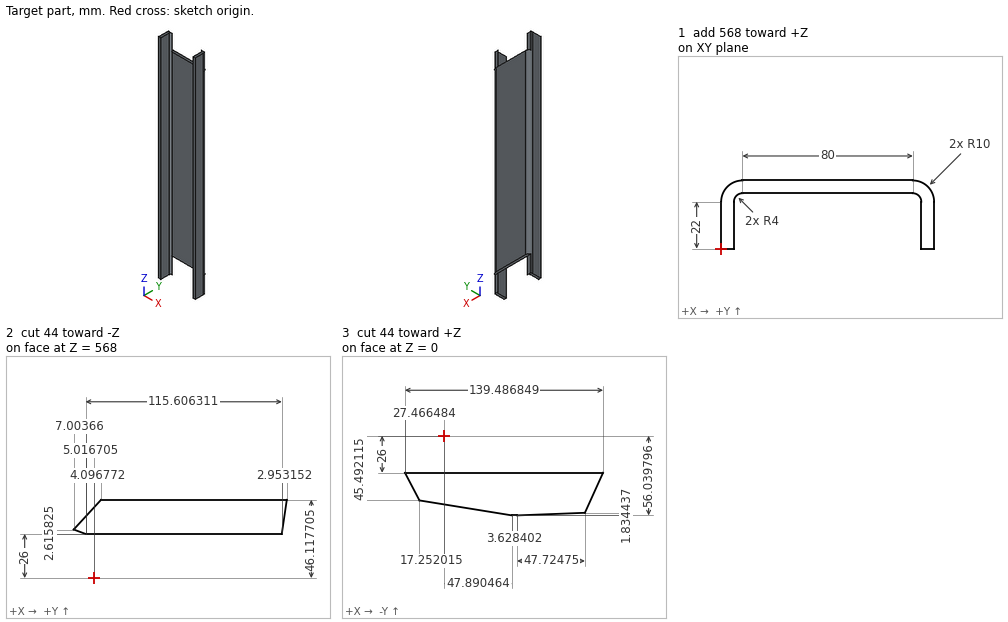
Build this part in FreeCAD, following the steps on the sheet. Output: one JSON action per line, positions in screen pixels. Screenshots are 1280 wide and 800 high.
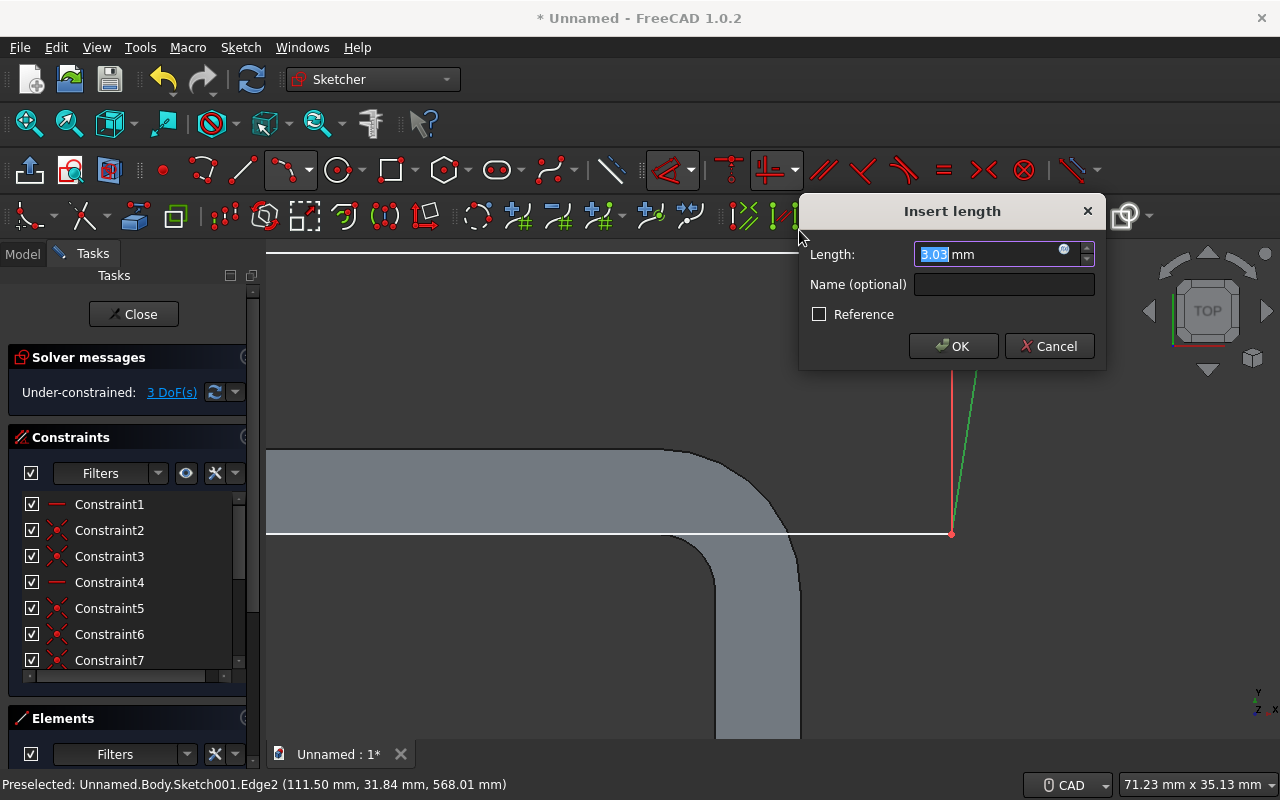
{"action": "type", "text": "2.953152"}
{"action": "key", "text": "Return"}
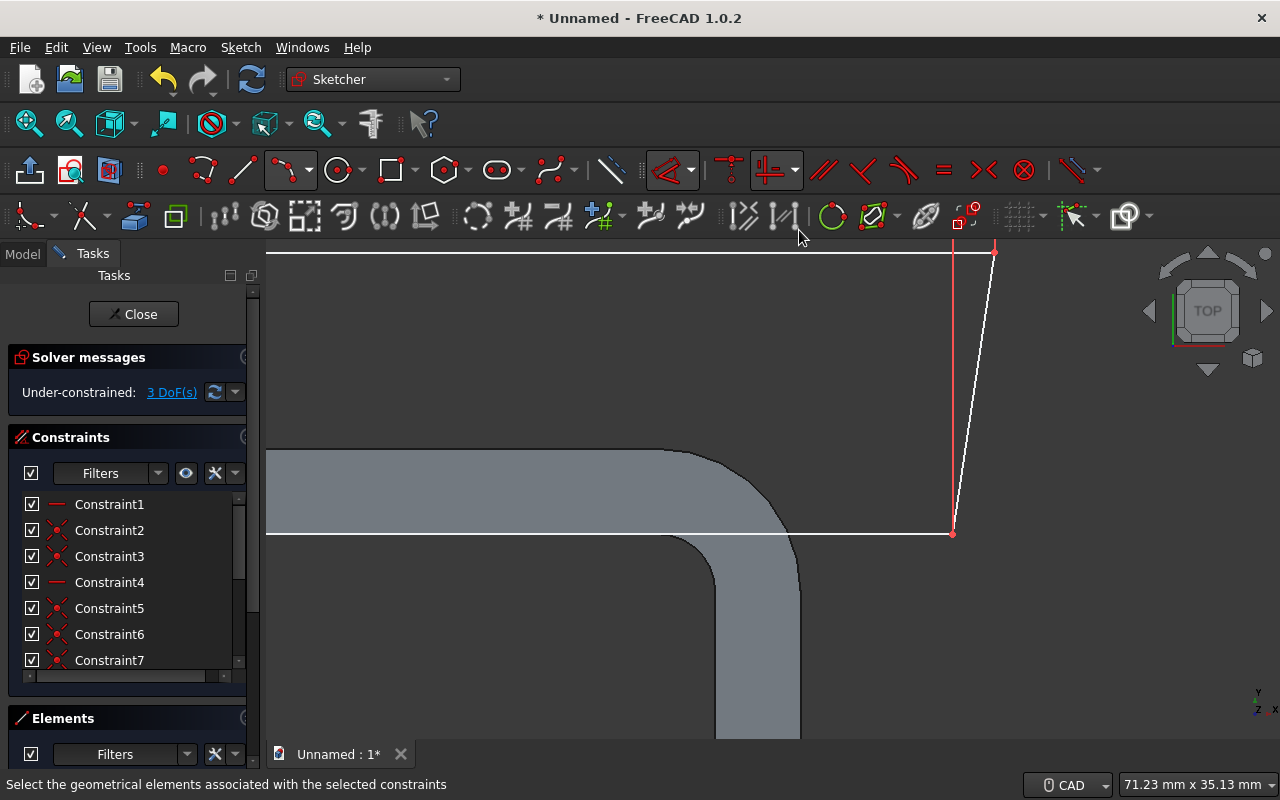
{"action": "scroll", "coordinate": [965, 451], "scroll_direction": "down", "scroll_amount": 6}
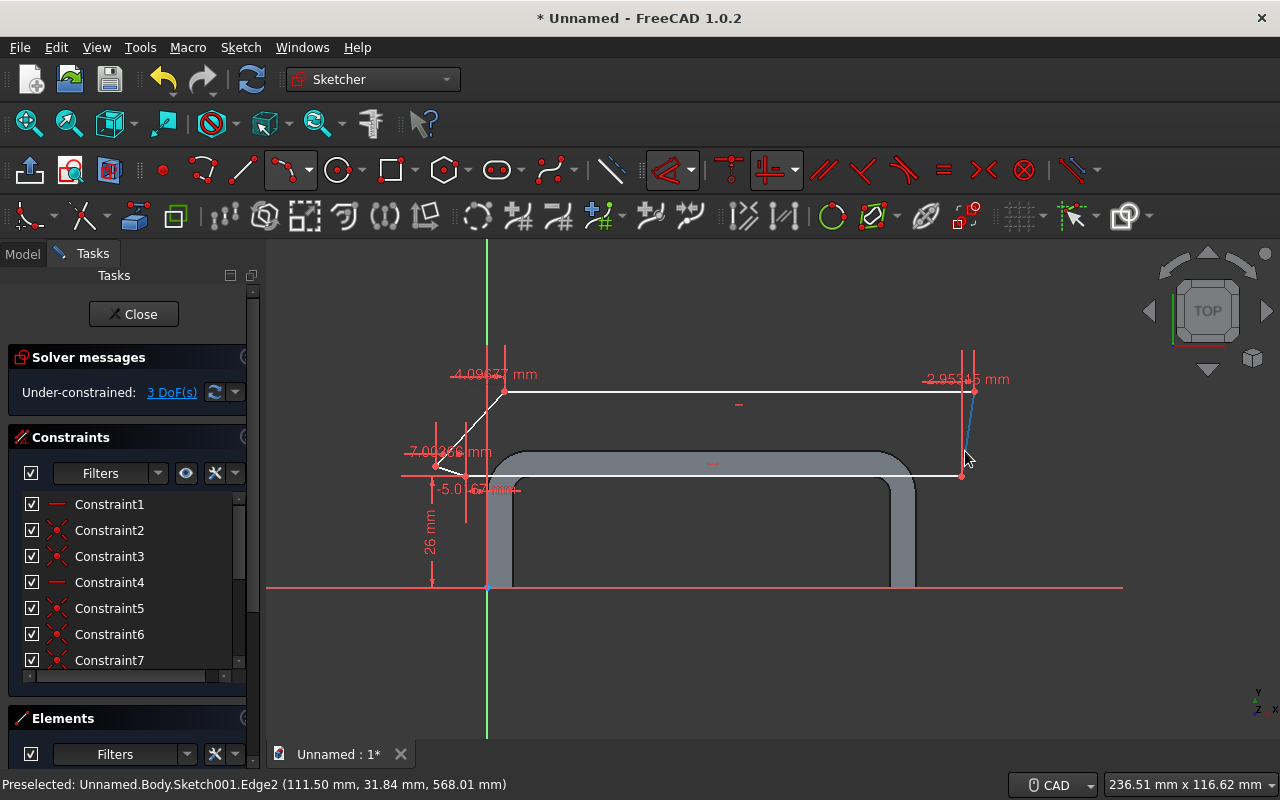
{"action": "scroll", "coordinate": [445, 469], "scroll_direction": "up", "scroll_amount": 7}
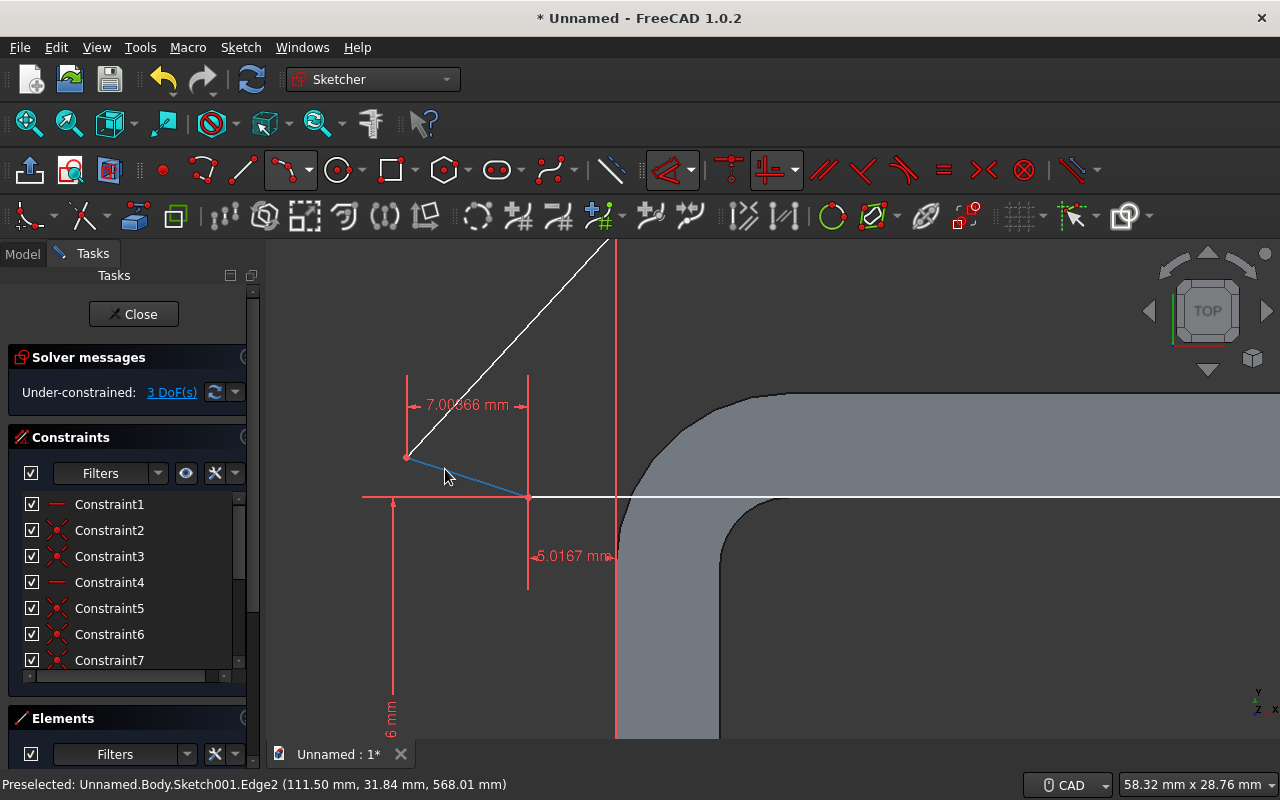
{"action": "left_click", "coordinate": [443, 470]}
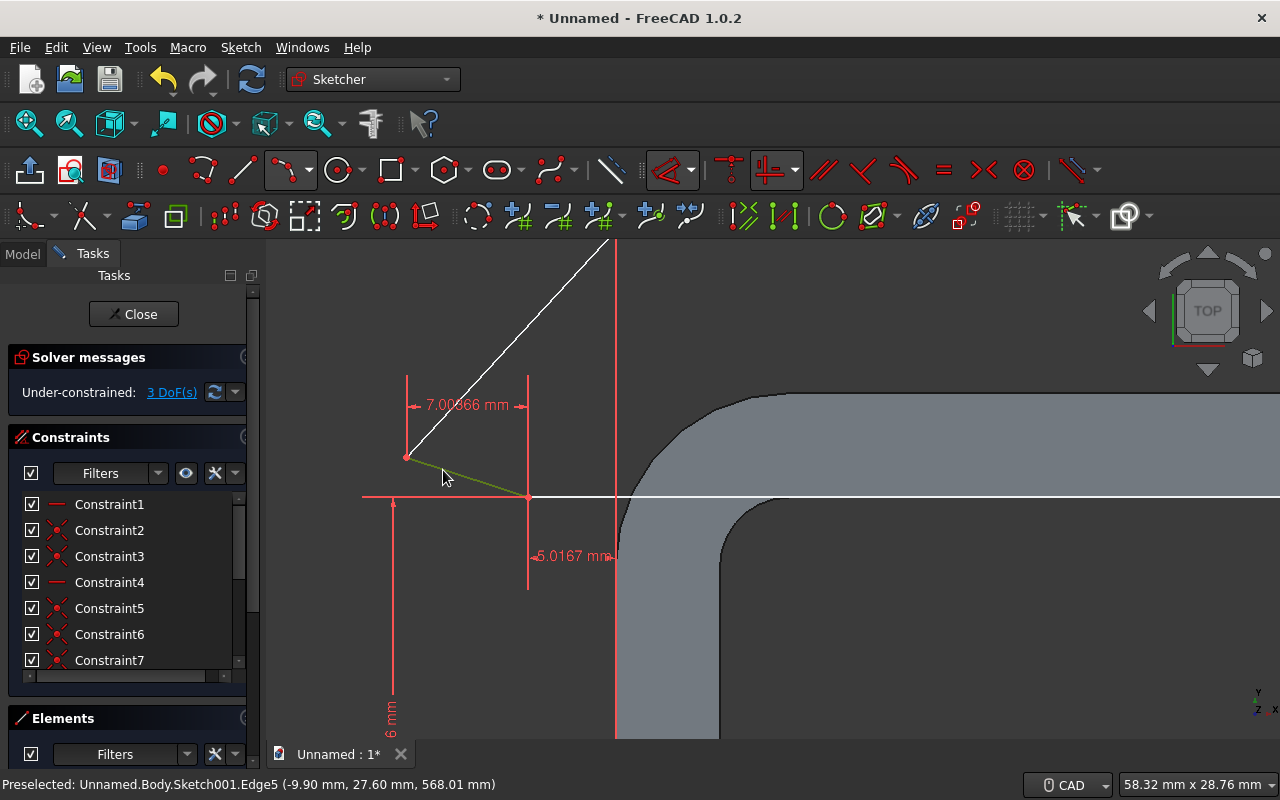
{"action": "left_click", "coordinate": [694, 170]}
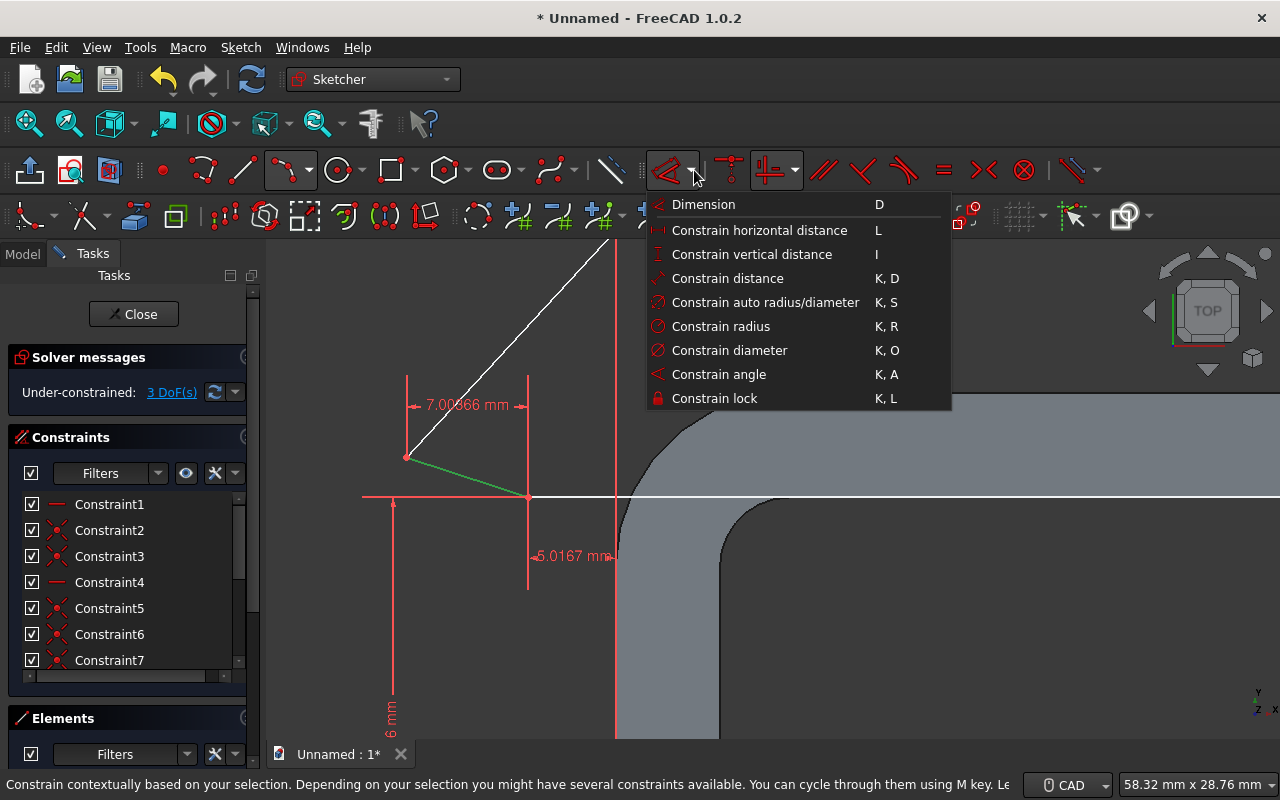
{"action": "left_click", "coordinate": [799, 254]}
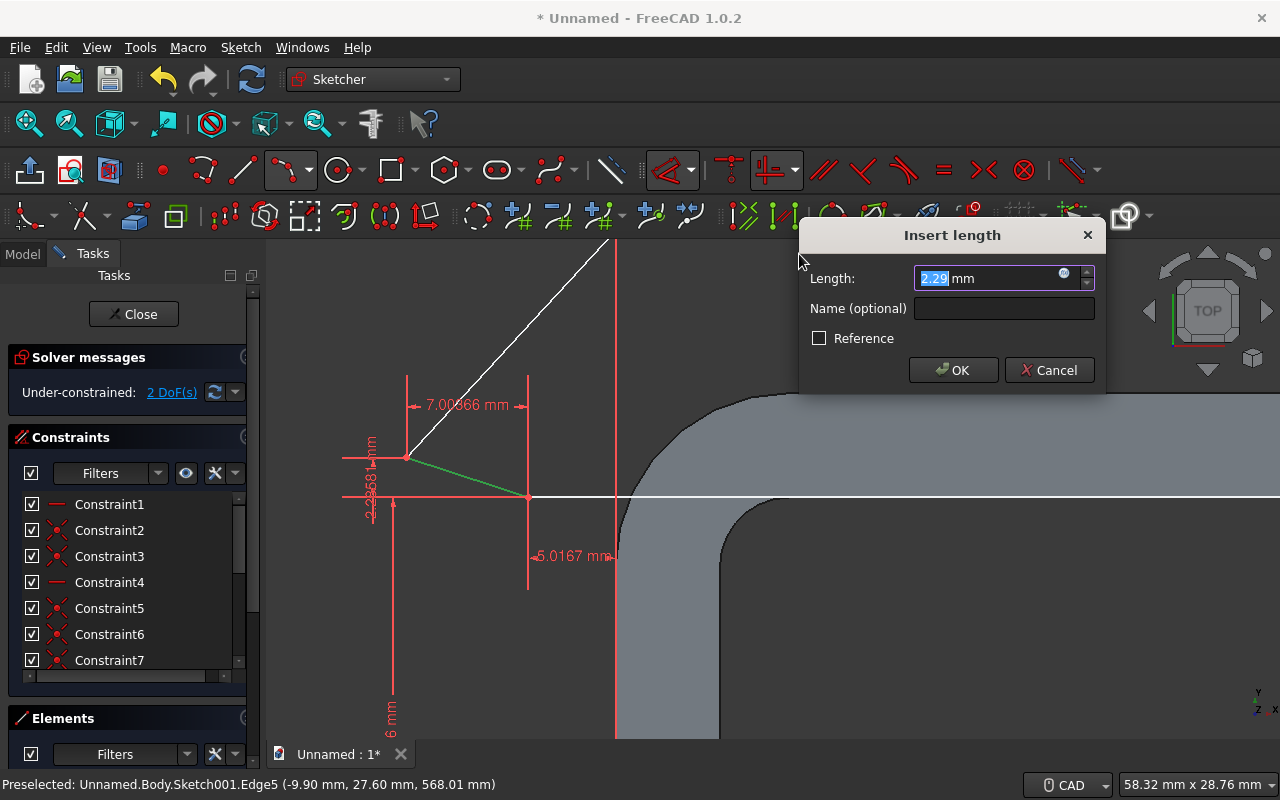
{"action": "type", "text": "2.615825"}
{"action": "key", "text": "Return"}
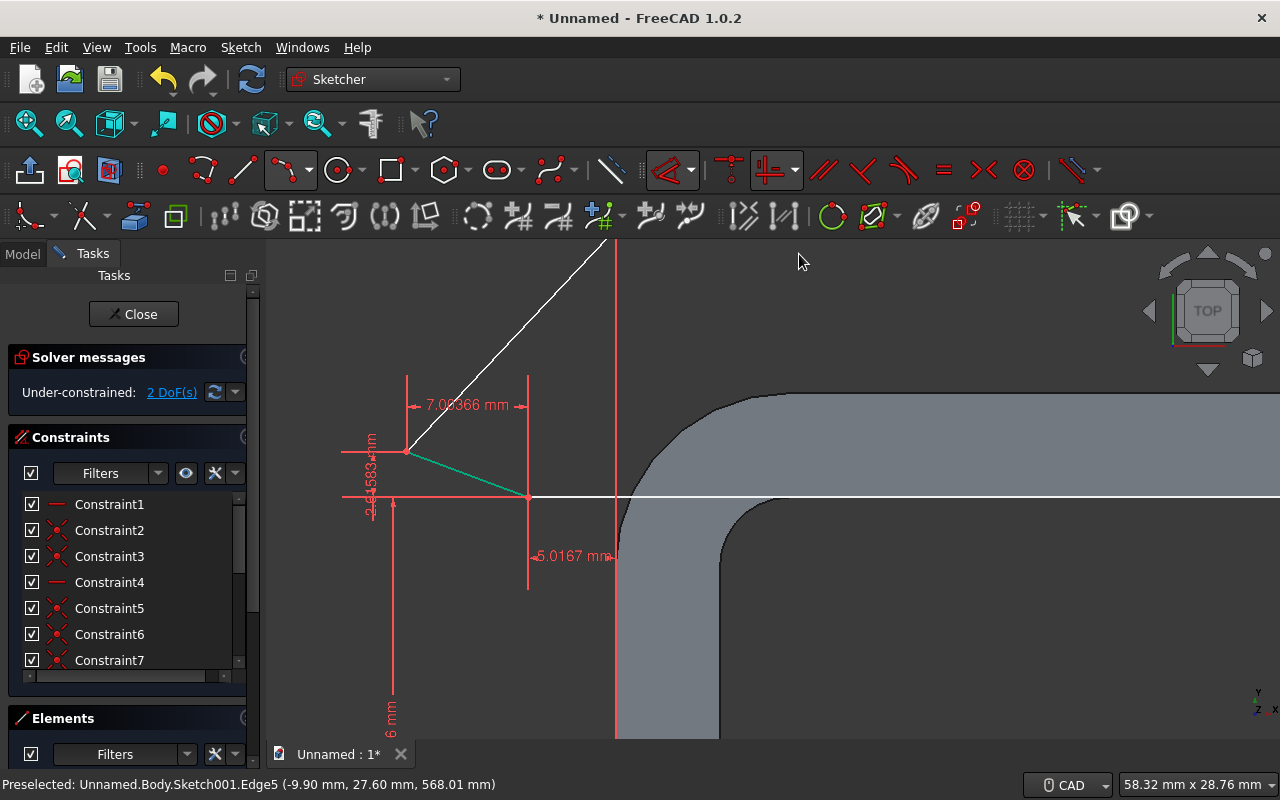
{"action": "scroll", "coordinate": [445, 470], "scroll_direction": "down", "scroll_amount": 7}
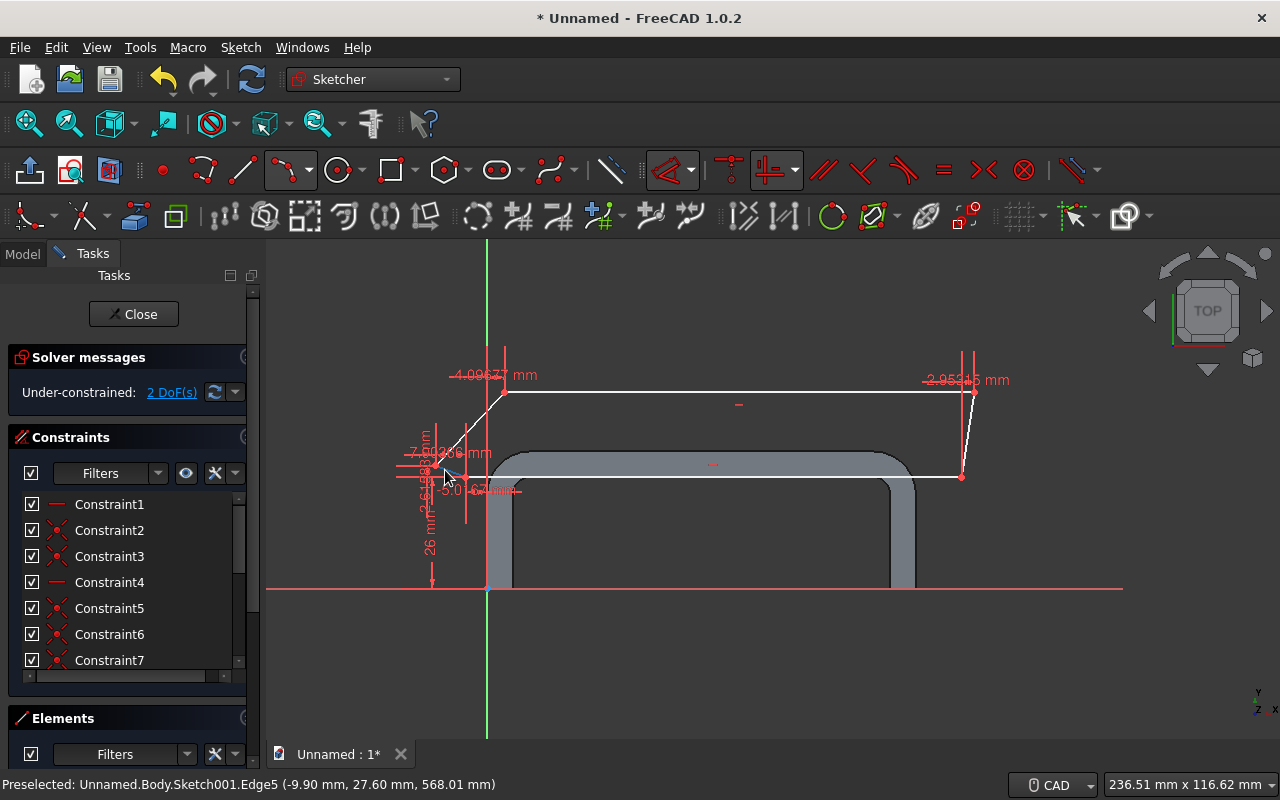
{"action": "left_click", "coordinate": [565, 477]}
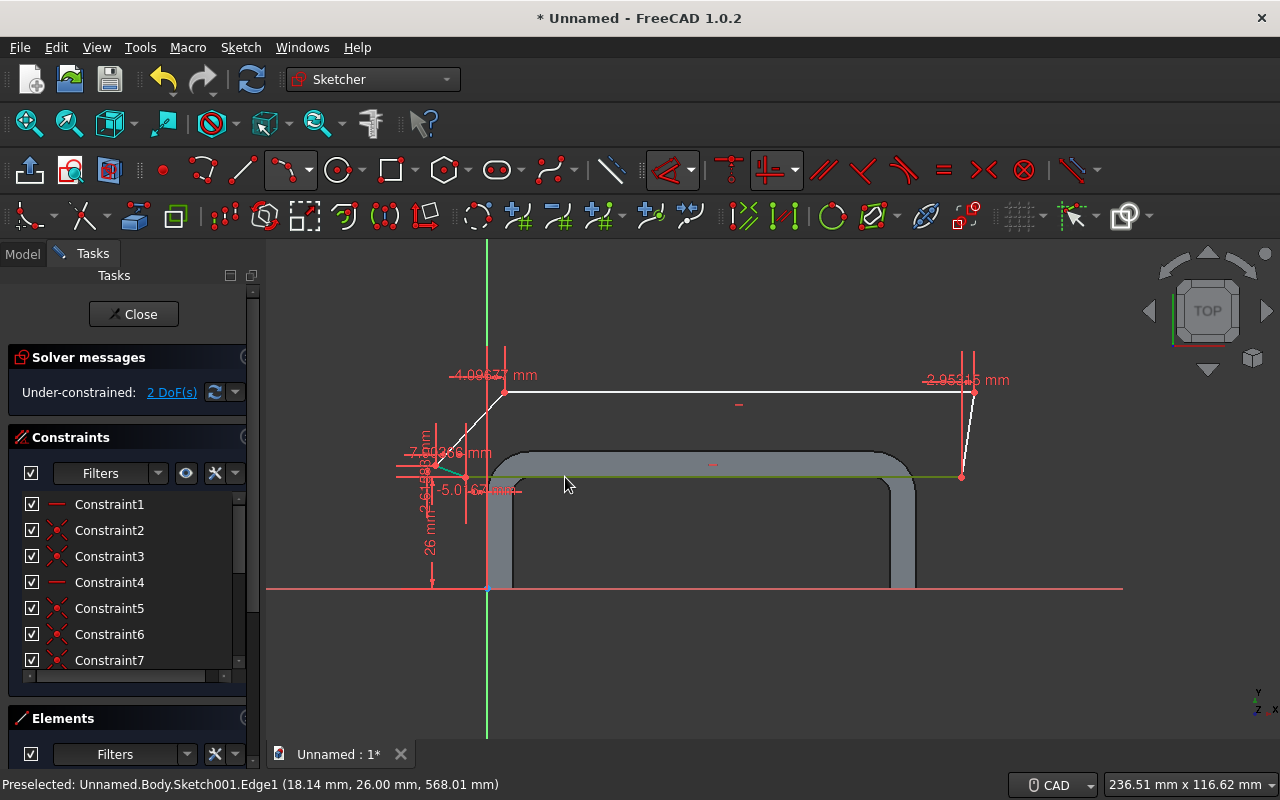
{"action": "key", "text": "l"}